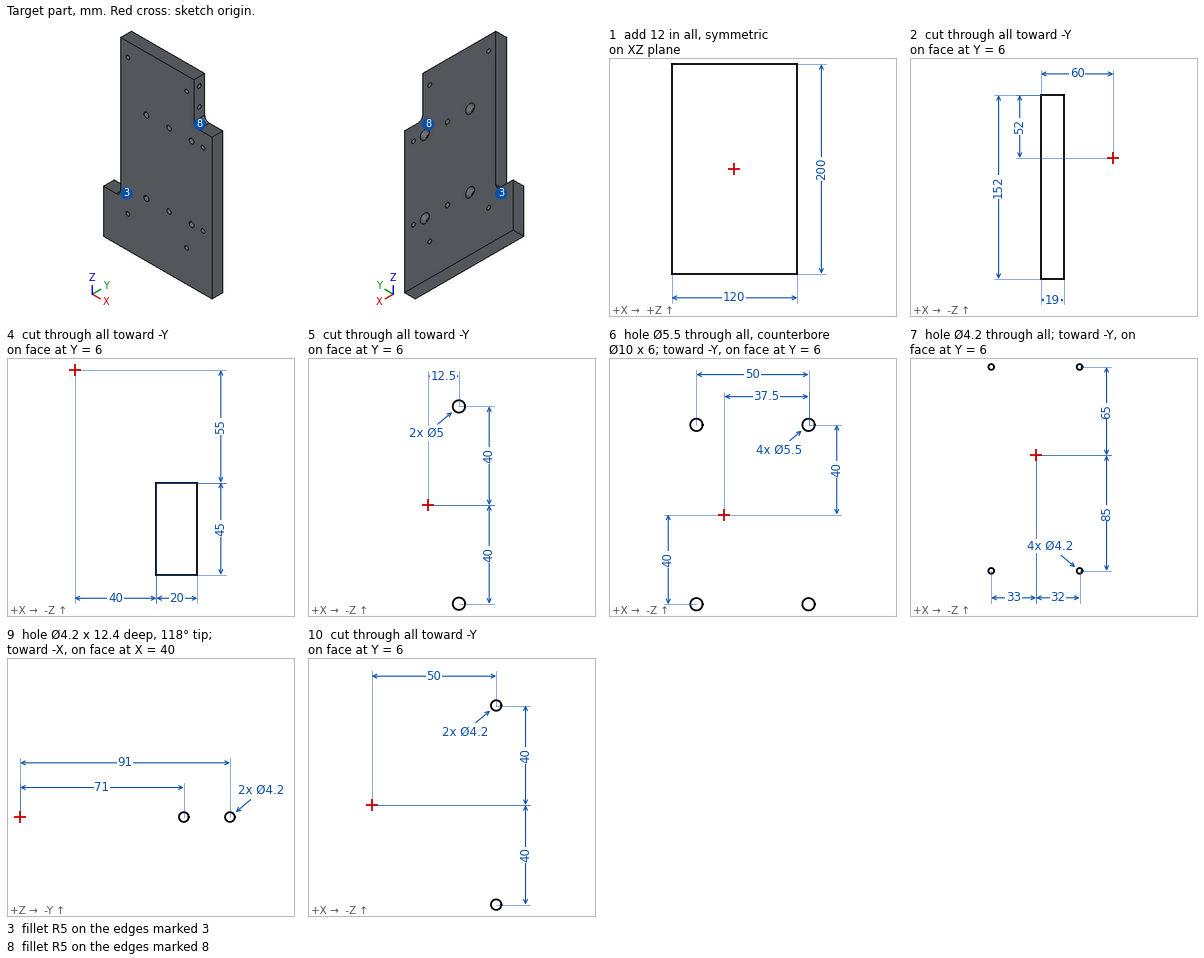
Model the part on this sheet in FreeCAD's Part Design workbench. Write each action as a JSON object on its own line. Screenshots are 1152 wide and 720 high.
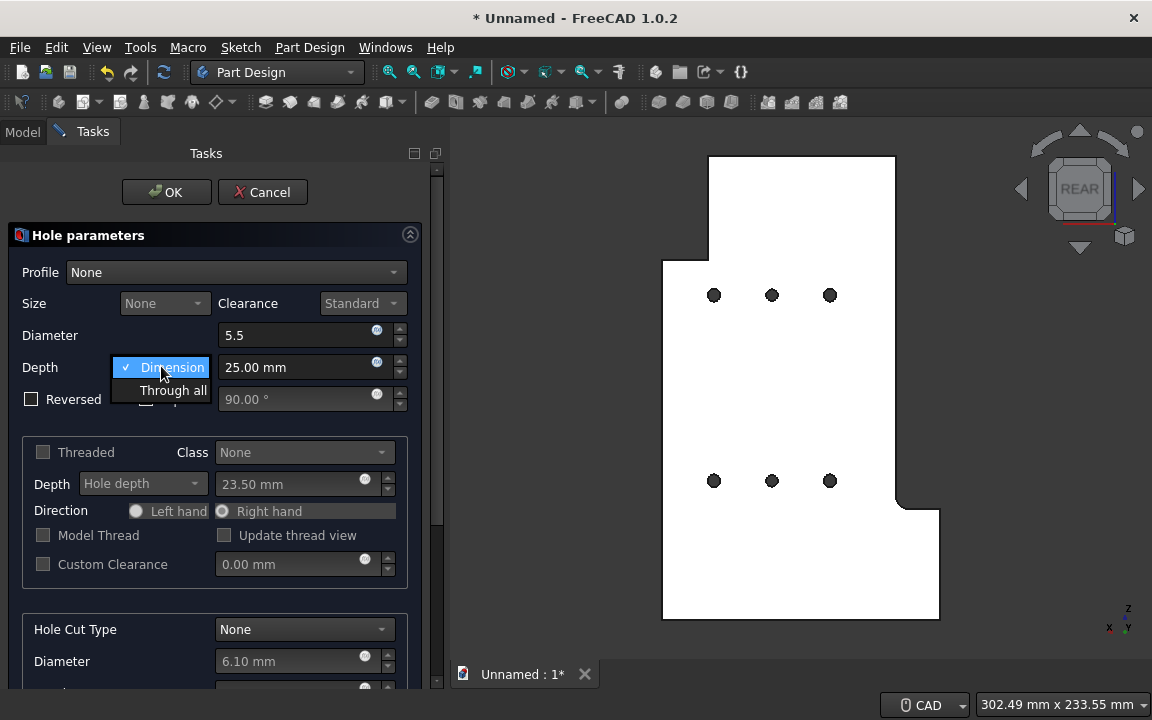
{"action": "left_click", "coordinate": [160, 390]}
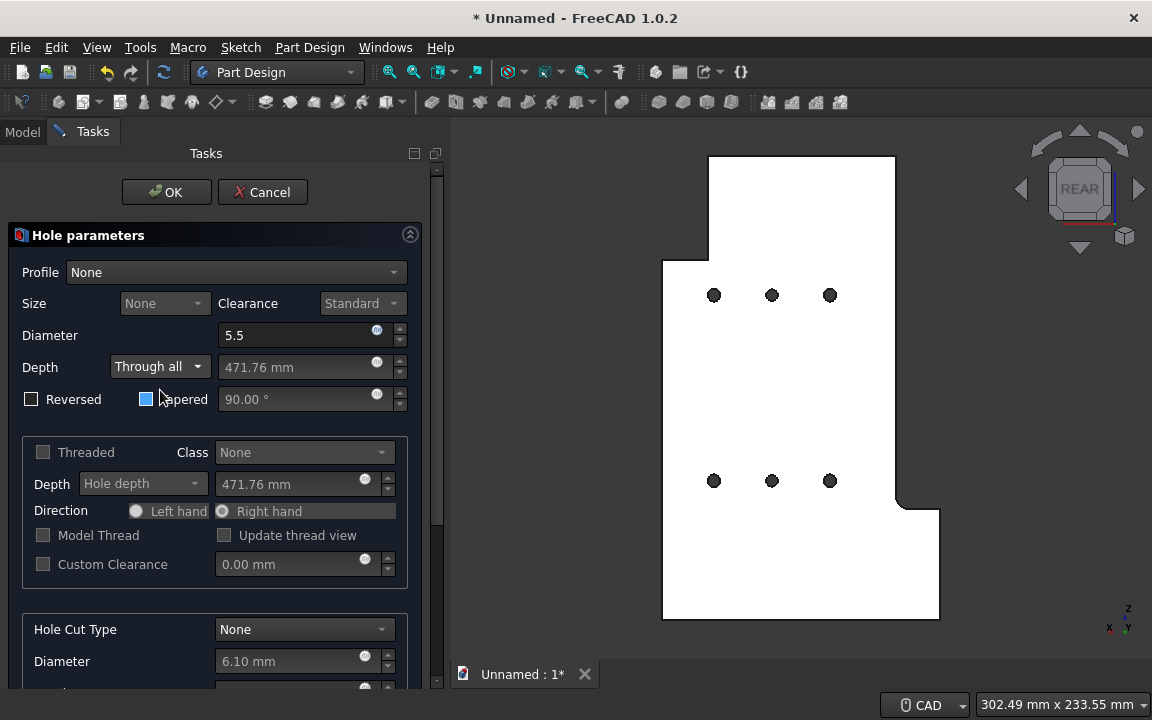
{"action": "left_click", "coordinate": [306, 630]}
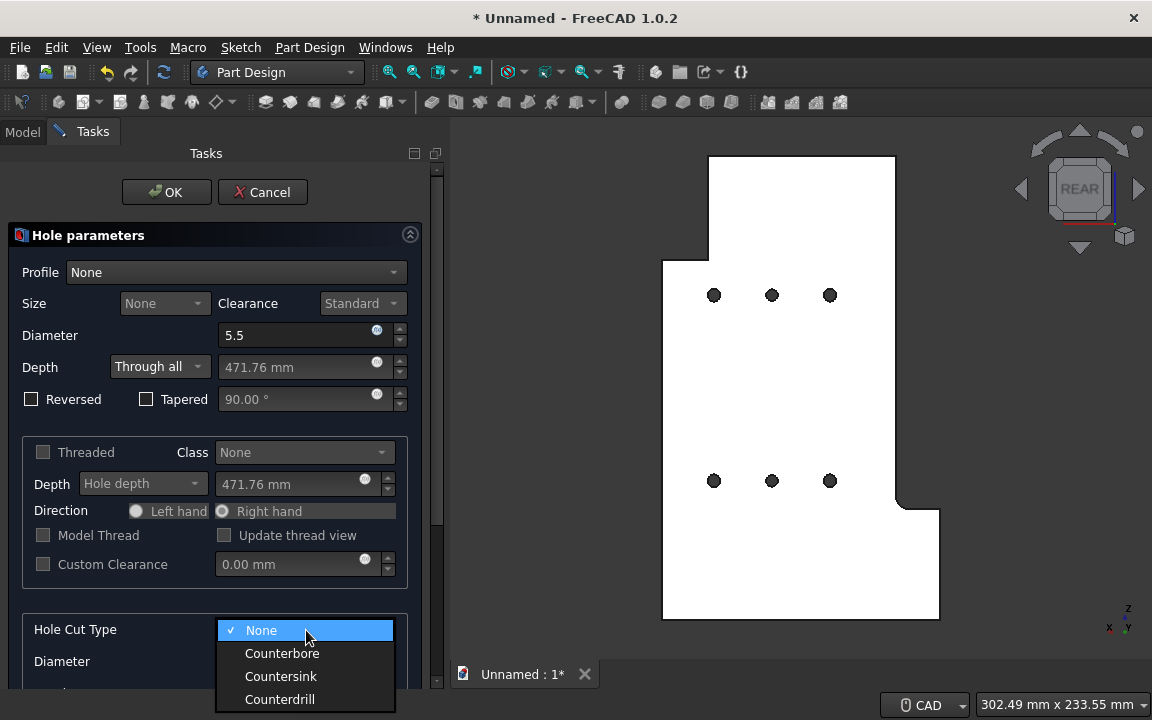
{"action": "left_click", "coordinate": [304, 654]}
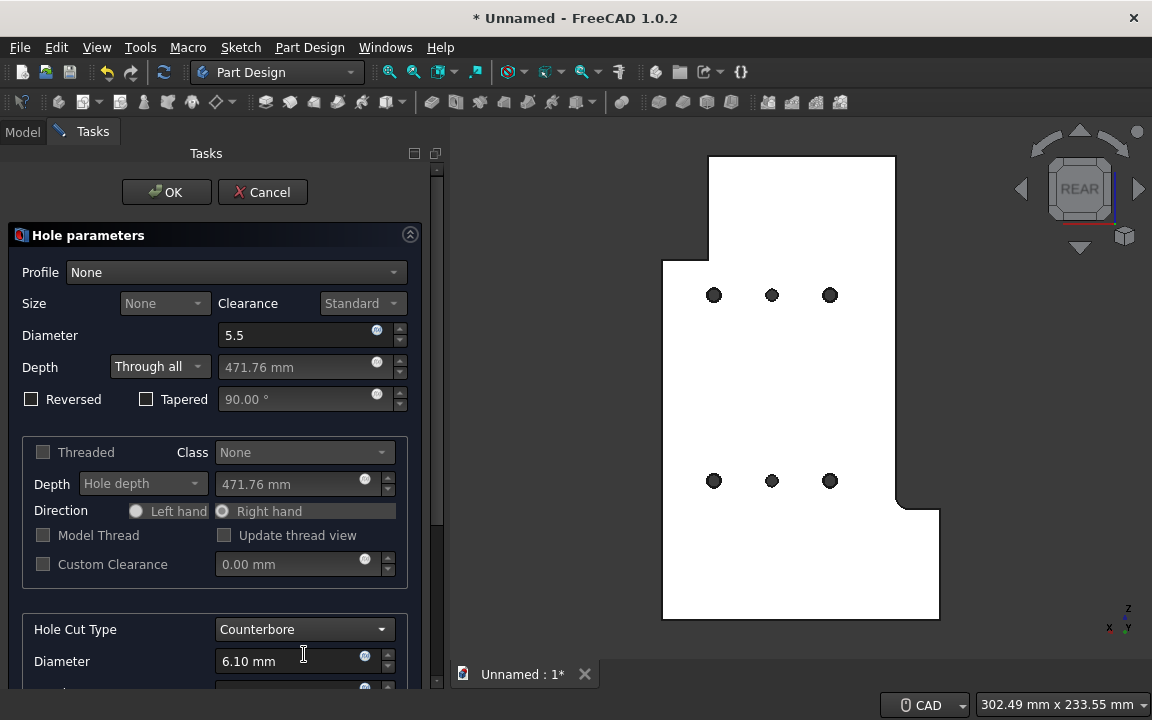
{"action": "triple_click", "coordinate": [298, 661]}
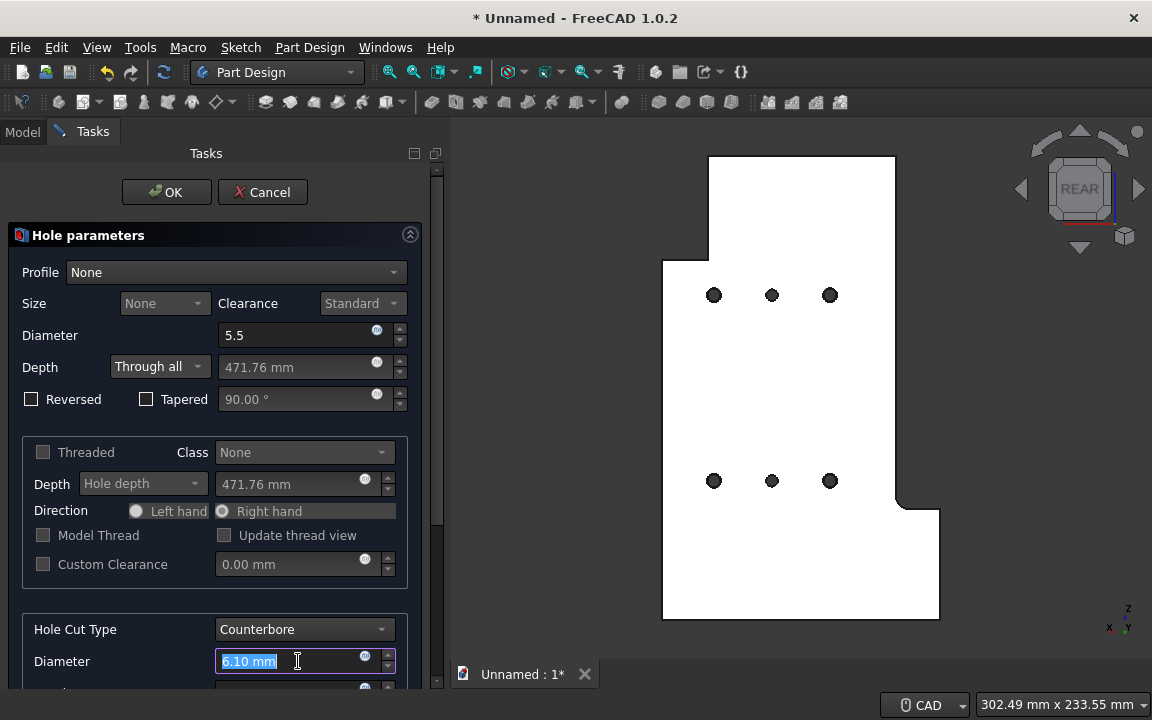
{"action": "type", "text": "10"}
{"action": "key", "text": "Tab"}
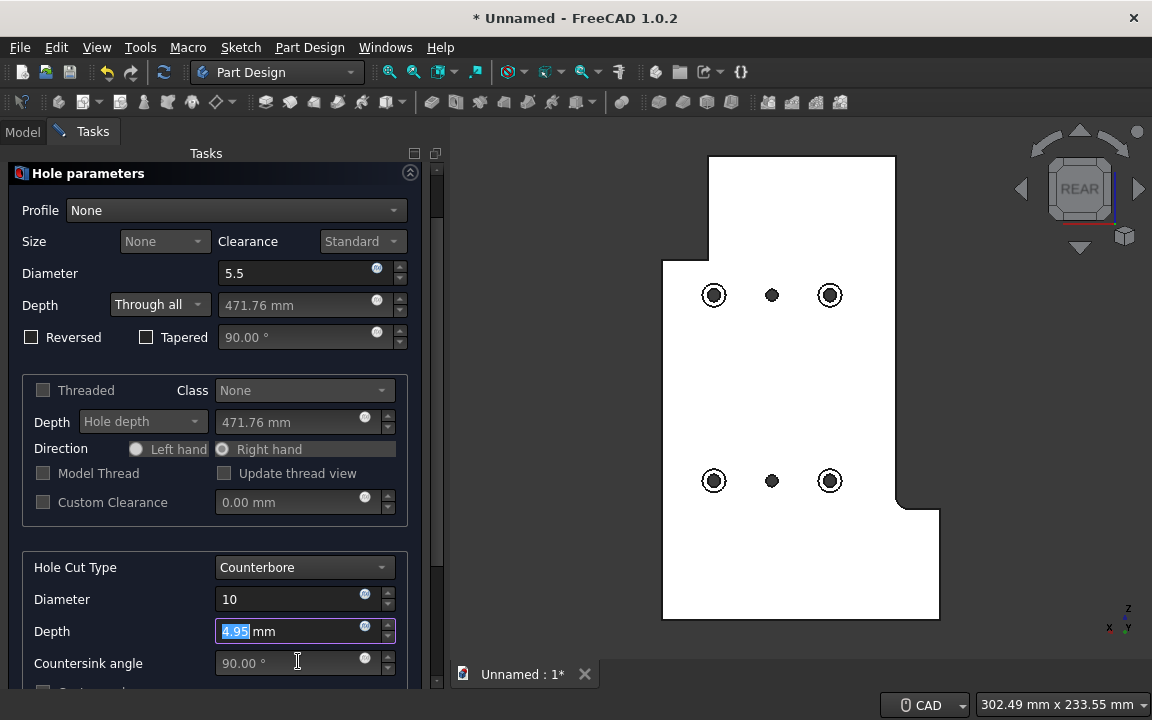
{"action": "type", "text": "6"}
{"action": "key", "text": "Tab"}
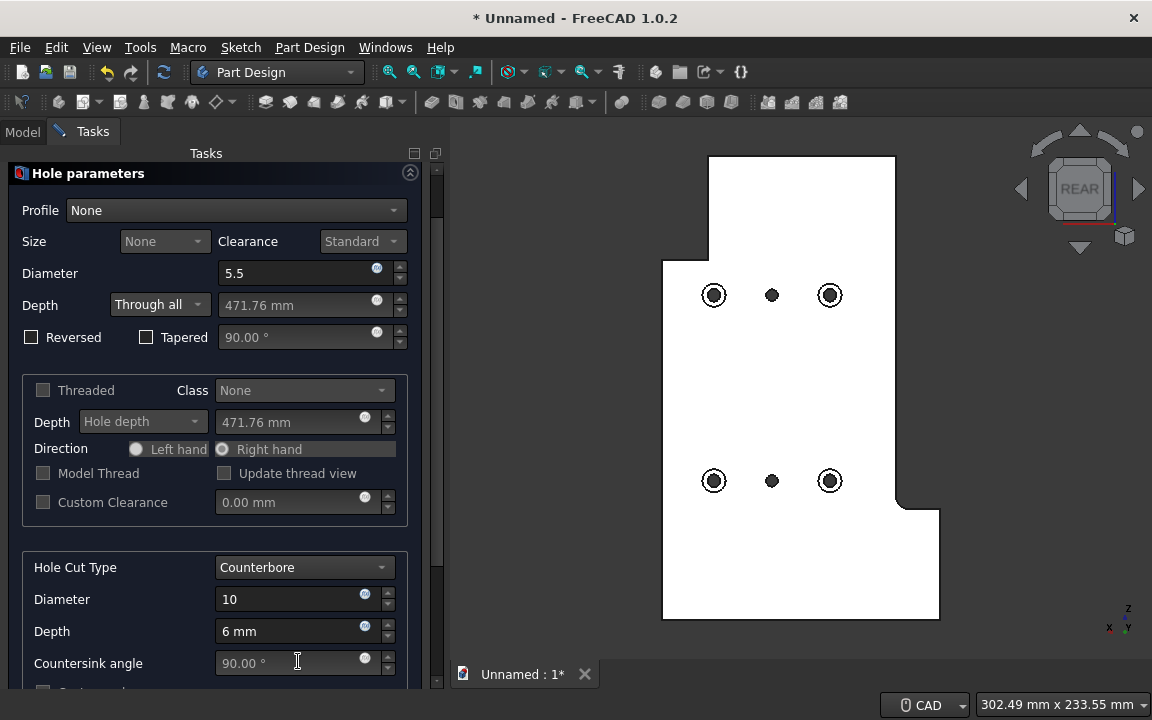
{"action": "scroll", "coordinate": [437, 426], "scroll_direction": "up", "scroll_amount": 2}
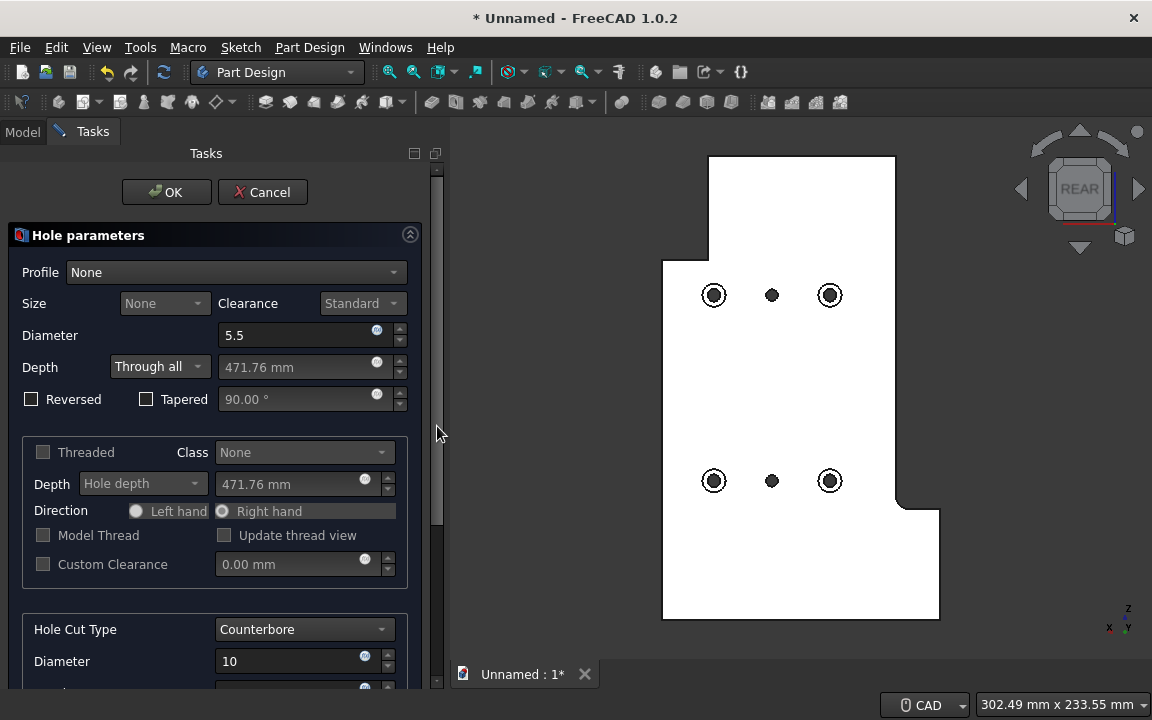
{"action": "left_click", "coordinate": [167, 192]}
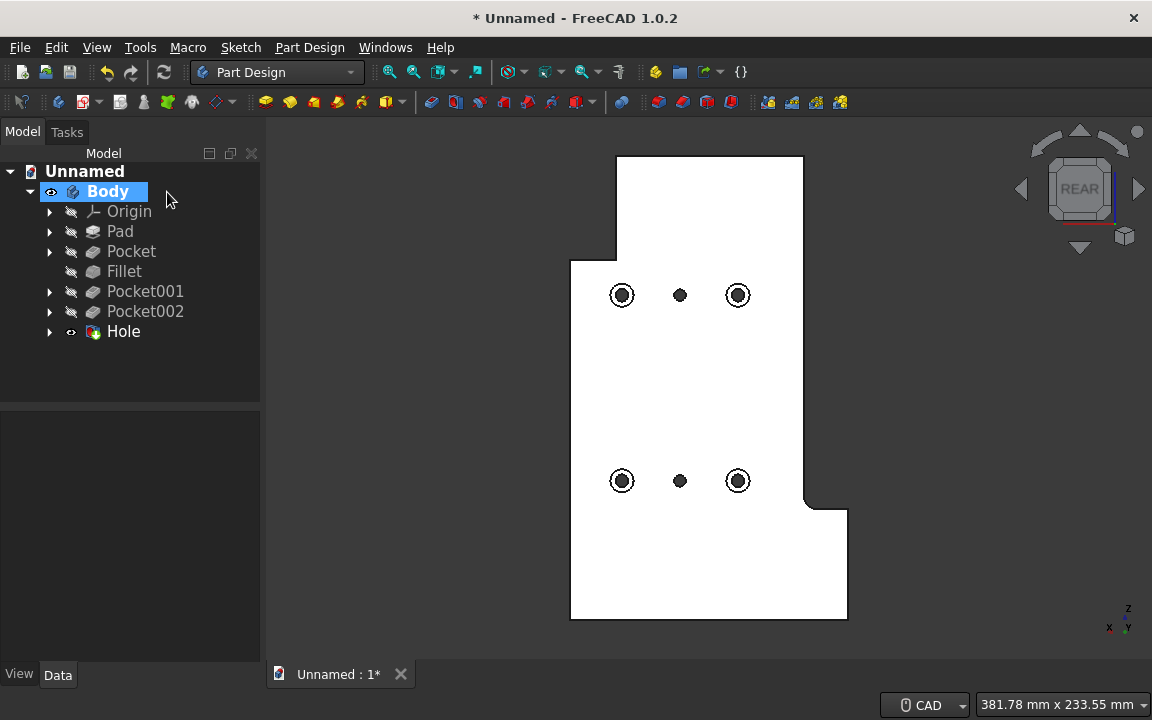
{"action": "left_click", "coordinate": [669, 387]}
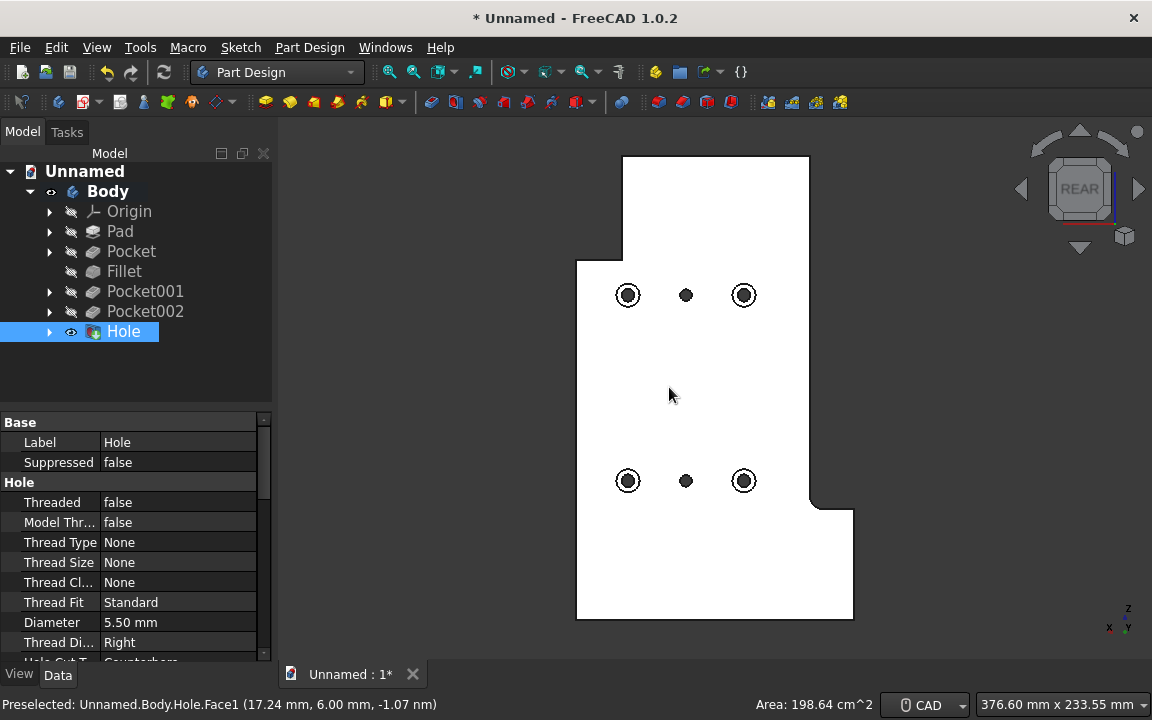
{"action": "left_click", "coordinate": [84, 102]}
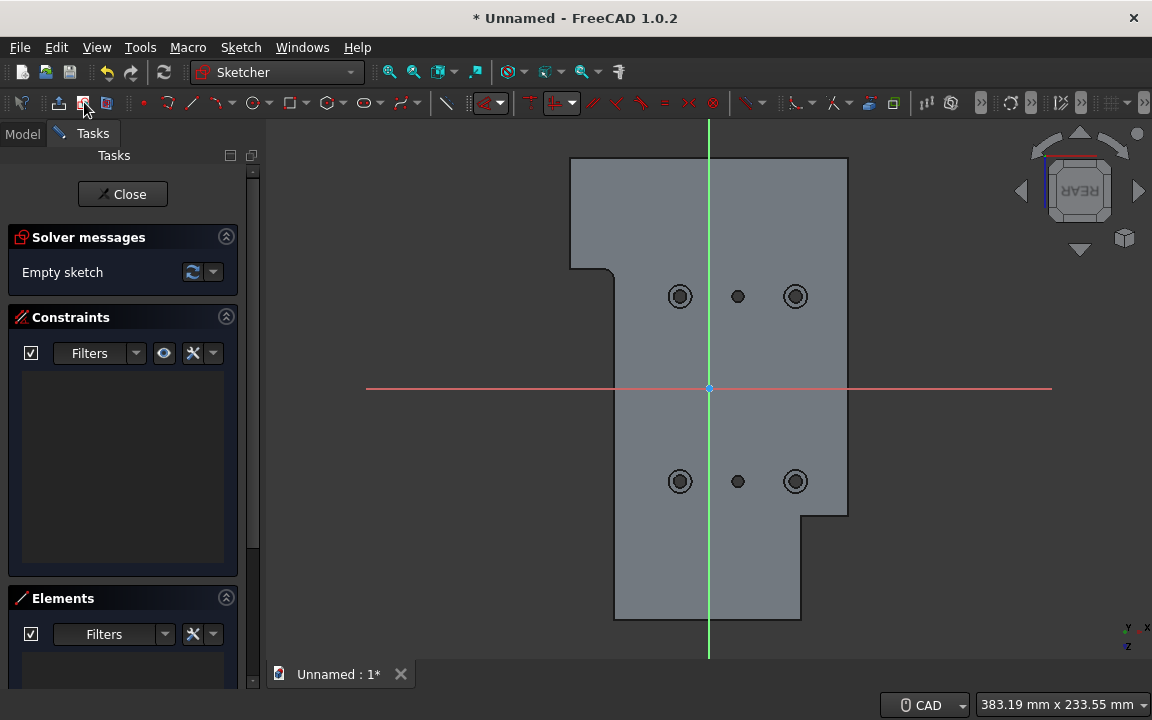
{"action": "left_click", "coordinate": [254, 104]}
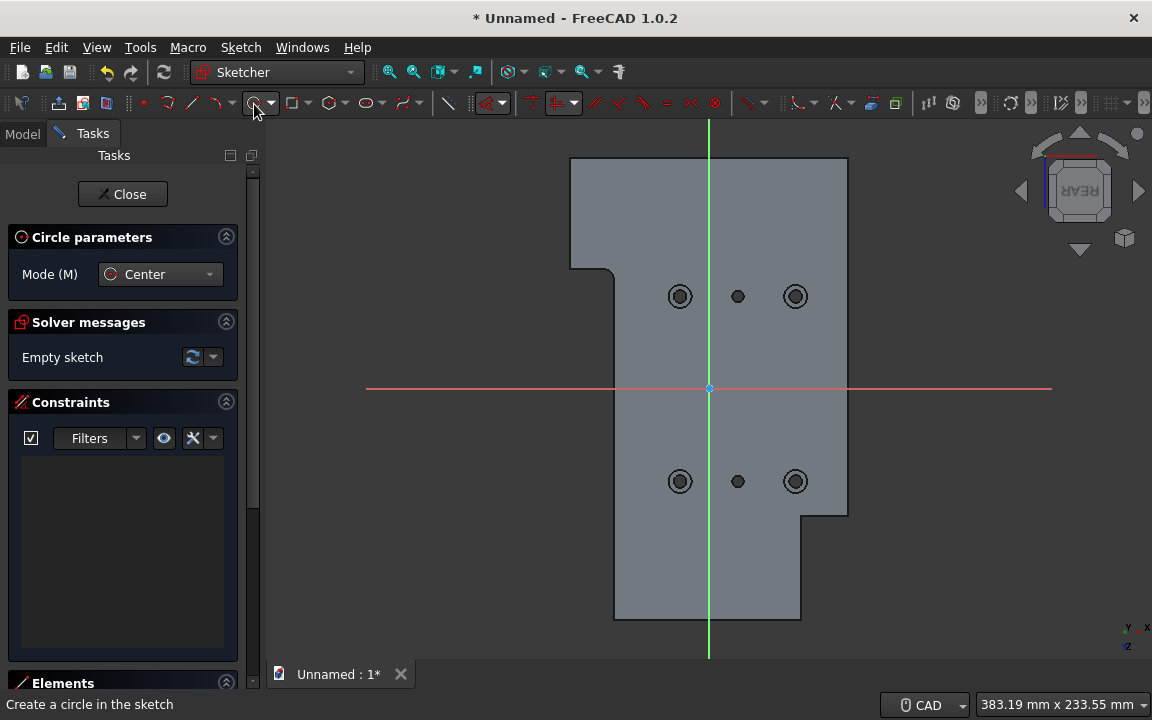
{"action": "scroll", "coordinate": [783, 586], "scroll_direction": "up", "scroll_amount": 8}